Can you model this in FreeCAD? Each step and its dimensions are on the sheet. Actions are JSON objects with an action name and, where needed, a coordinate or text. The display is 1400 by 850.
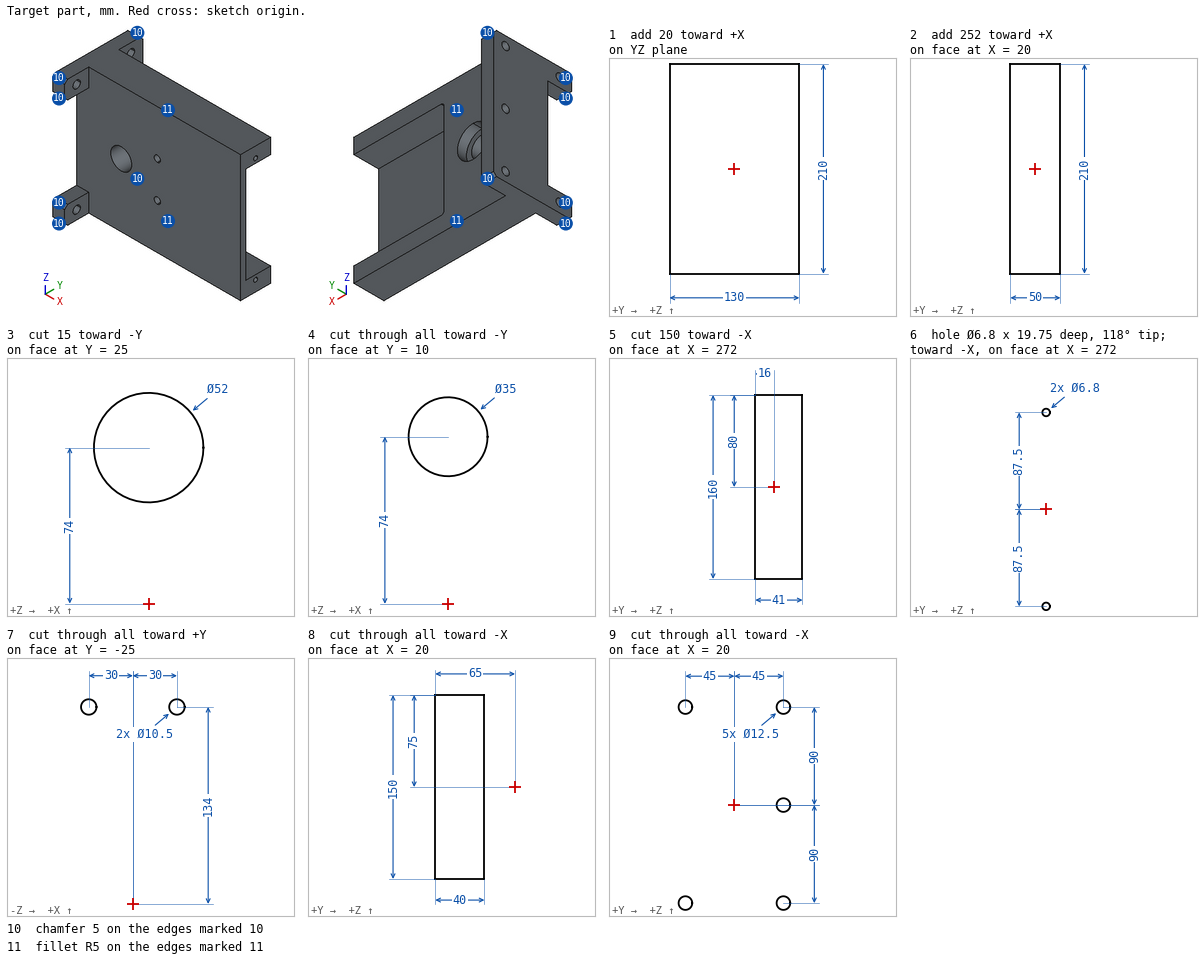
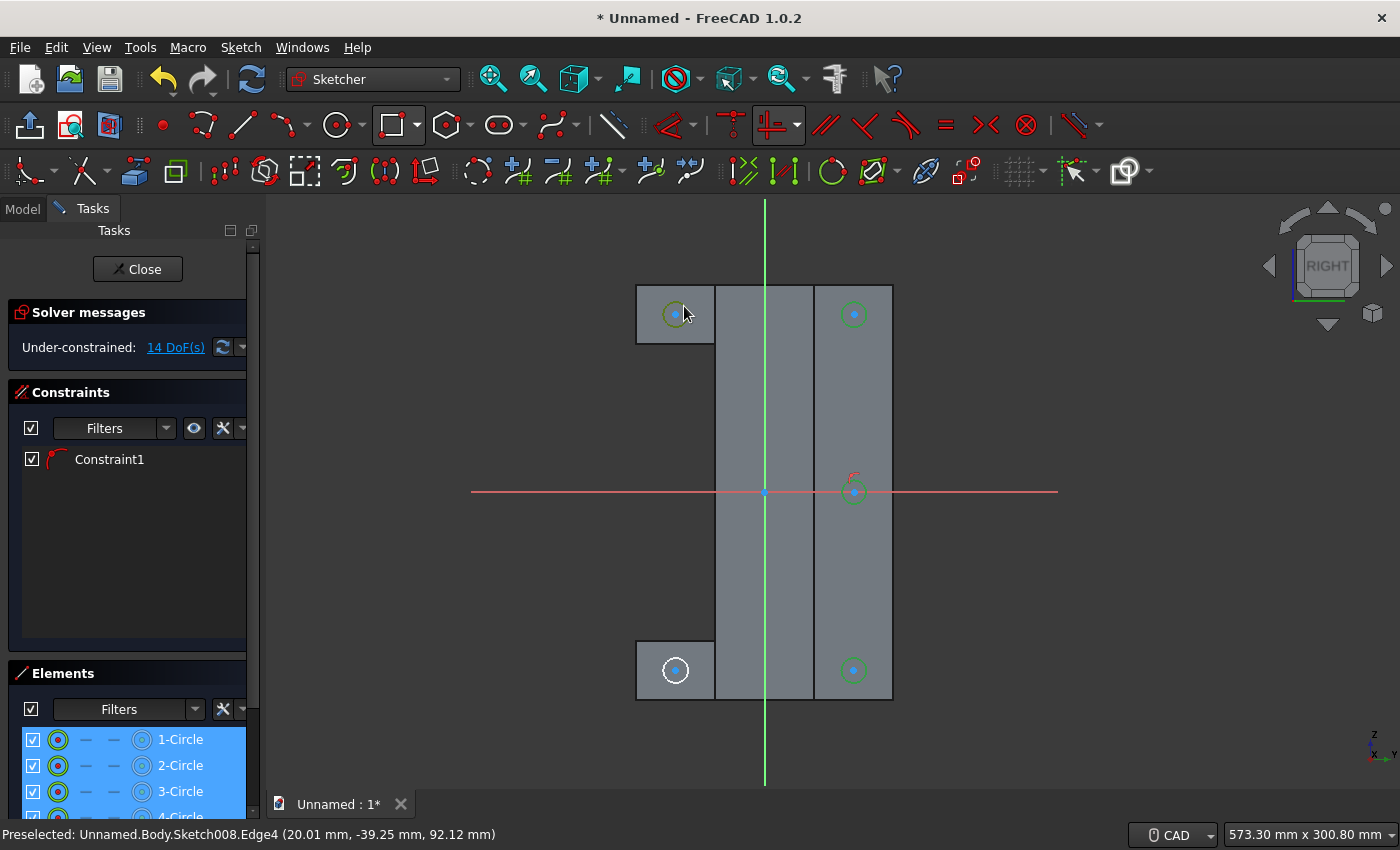
{"action": "left_click", "coordinate": [684, 662]}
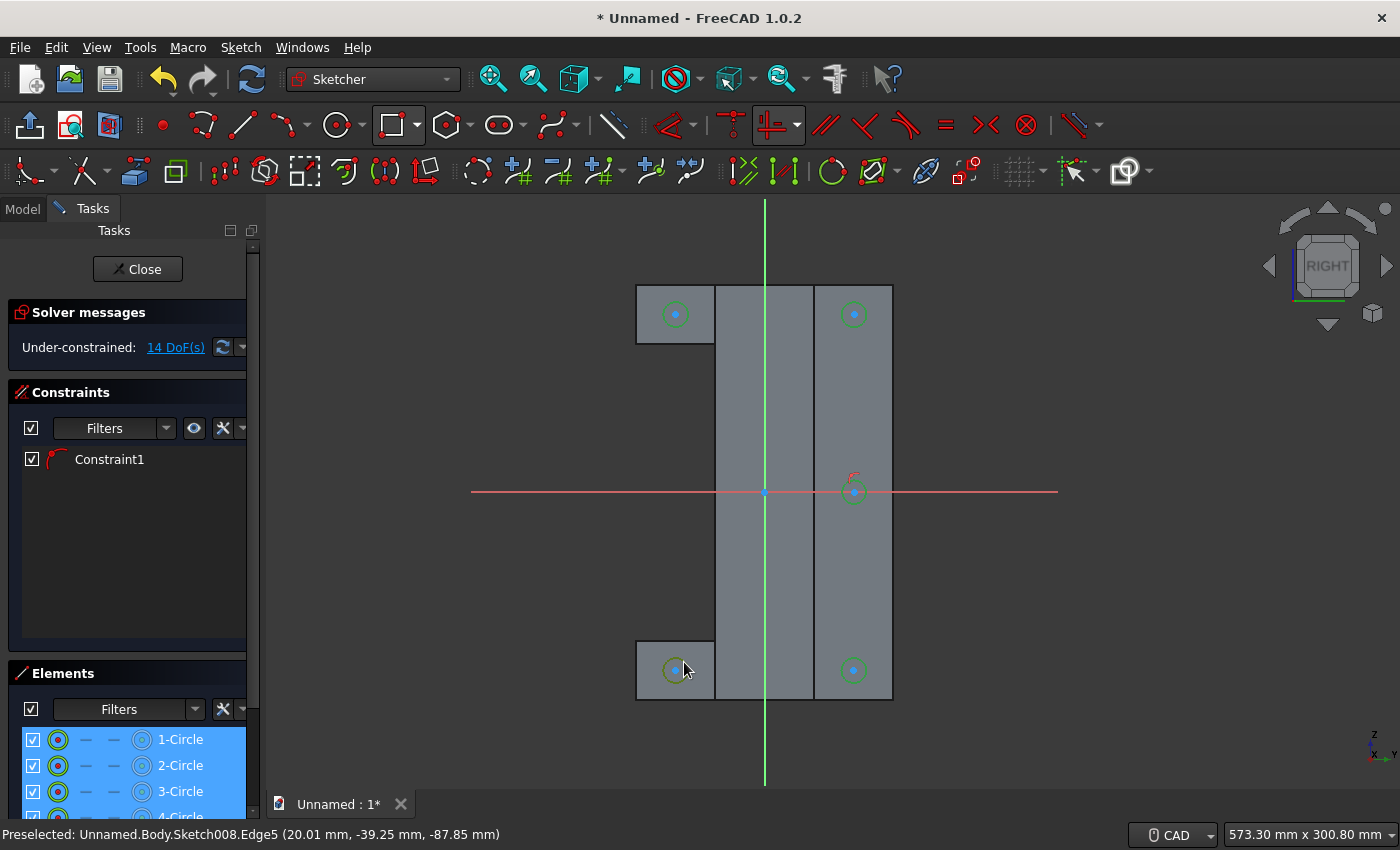
{"action": "left_click", "coordinate": [946, 126]}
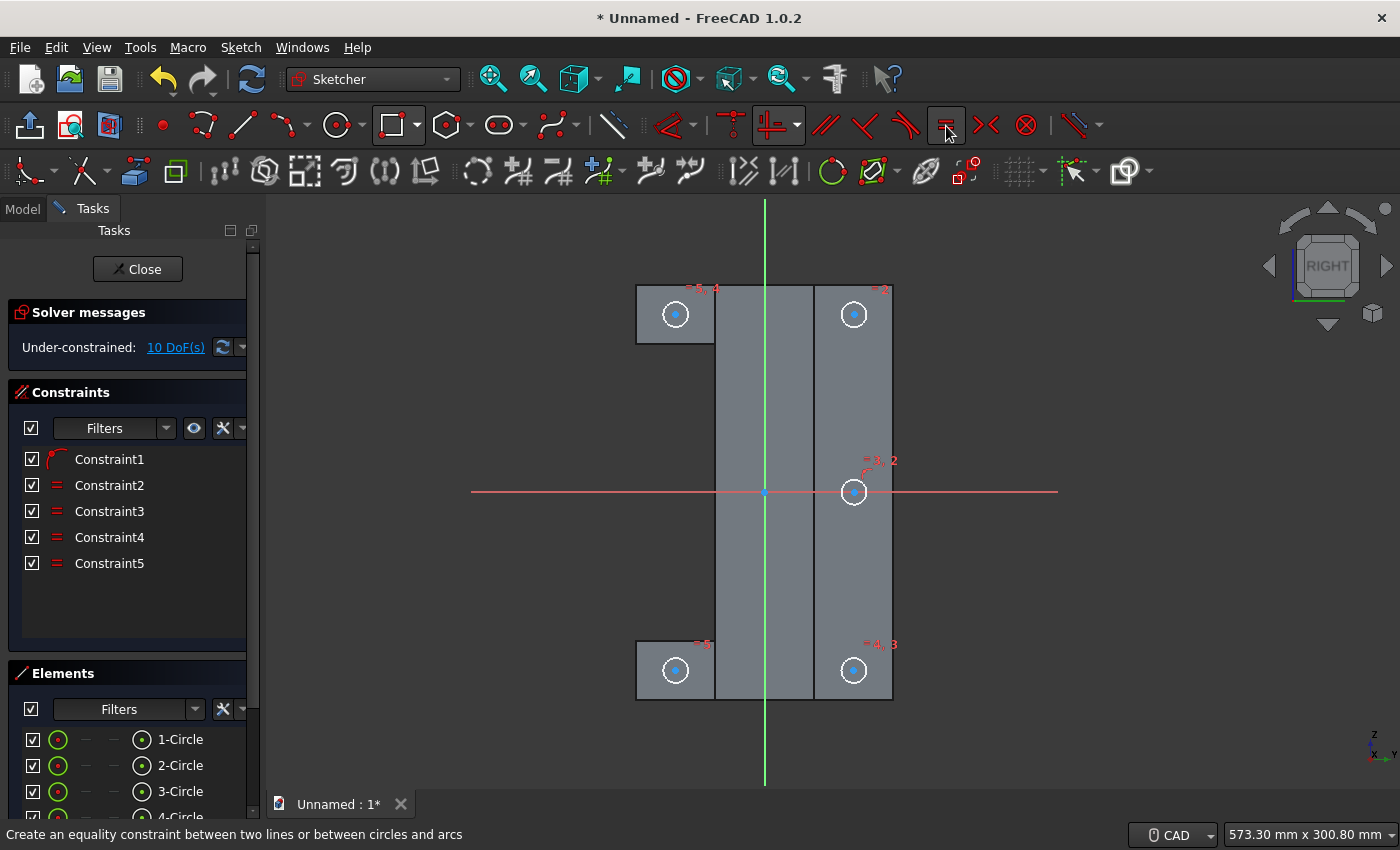
{"action": "left_click", "coordinate": [854, 315]}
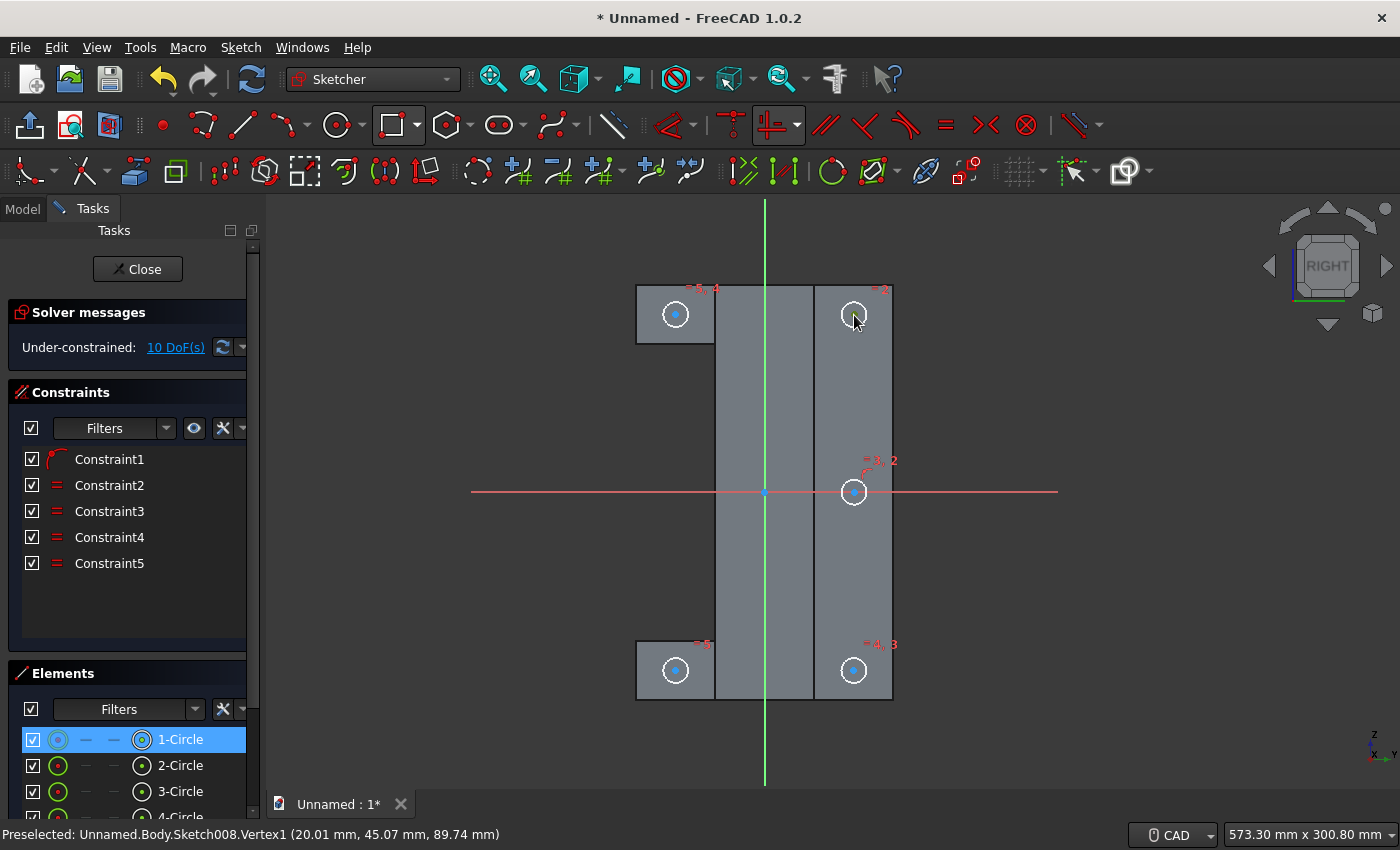
{"action": "left_click", "coordinate": [854, 492]}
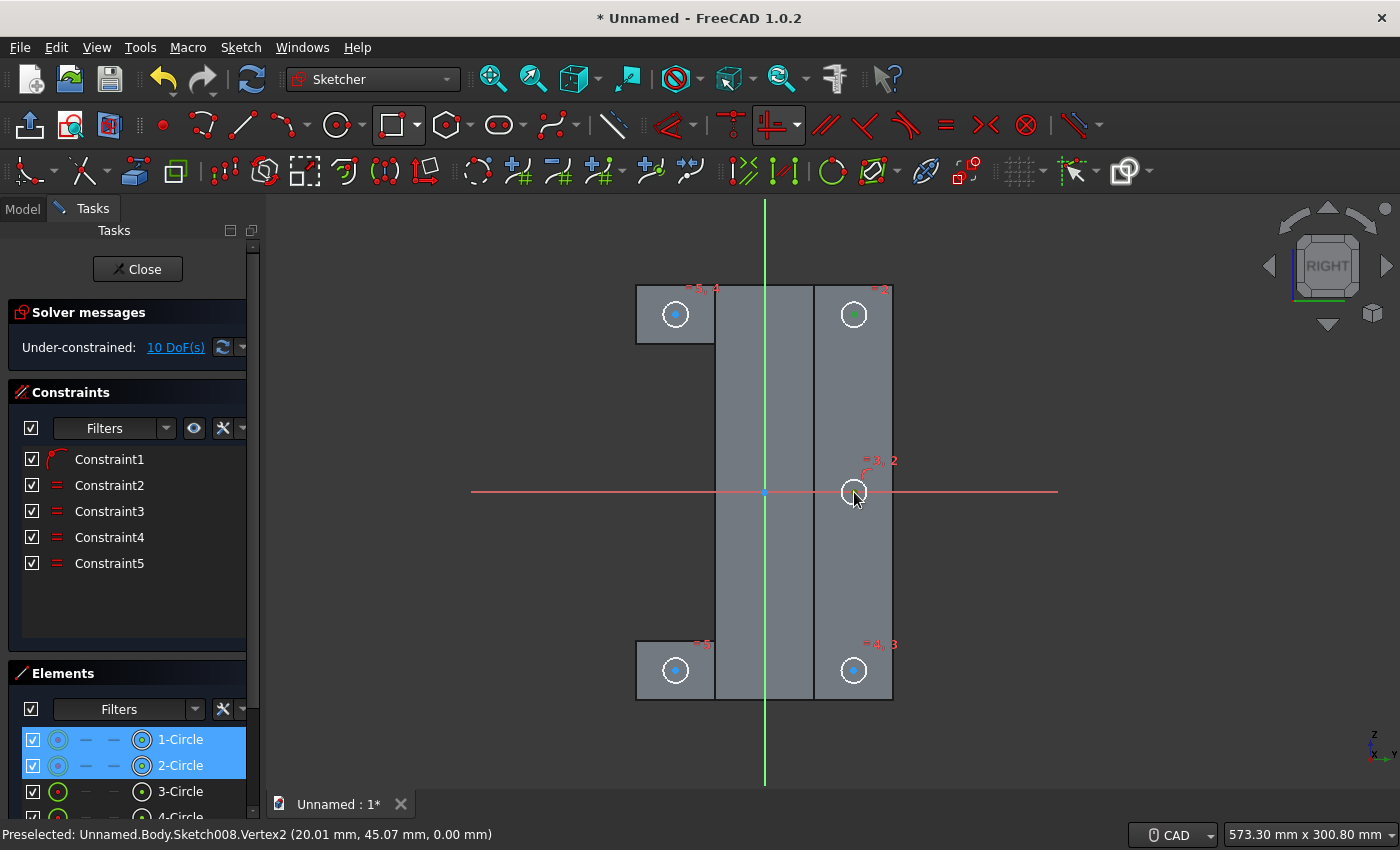
{"action": "key", "text": "v"}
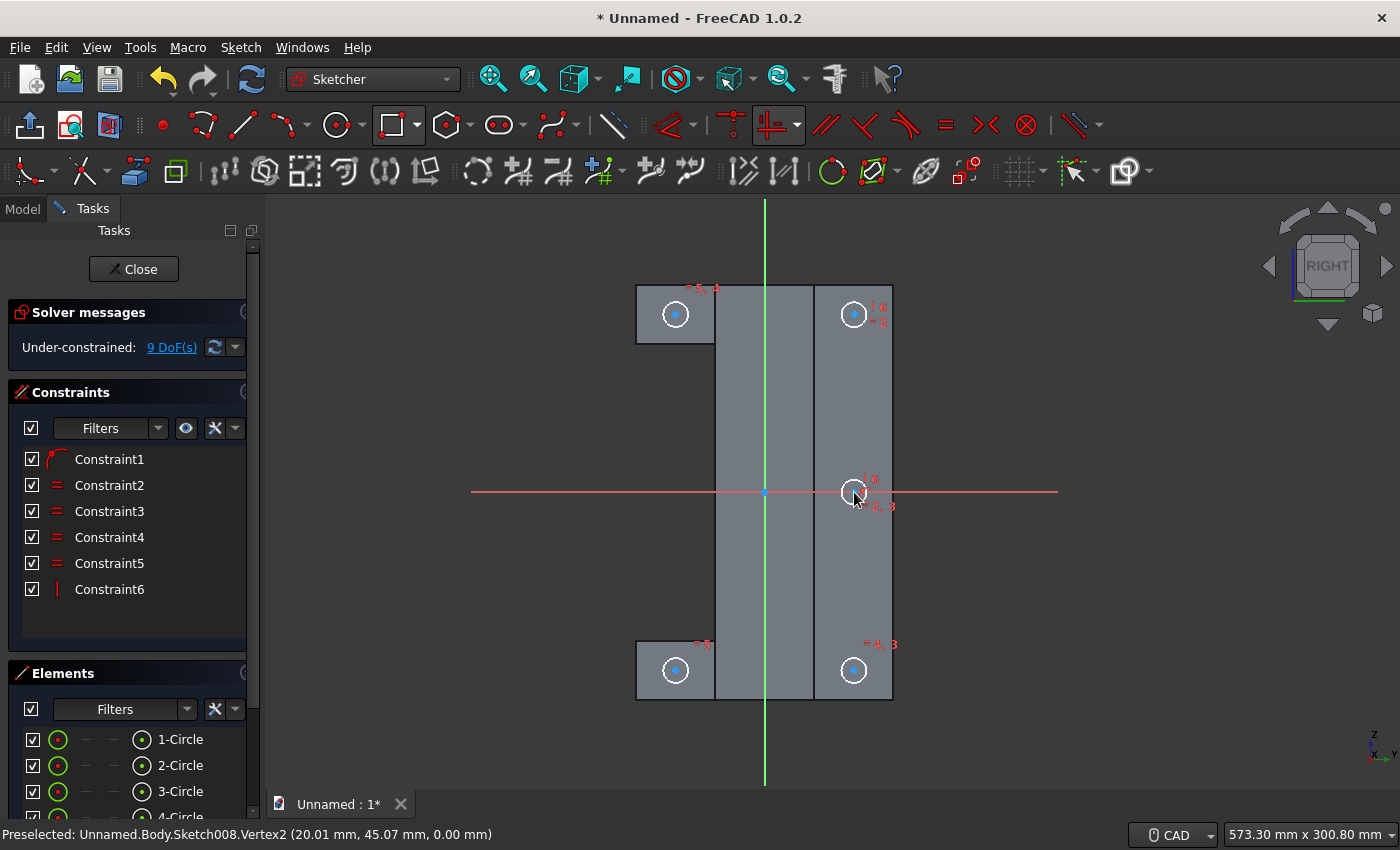
{"action": "left_click", "coordinate": [854, 492]}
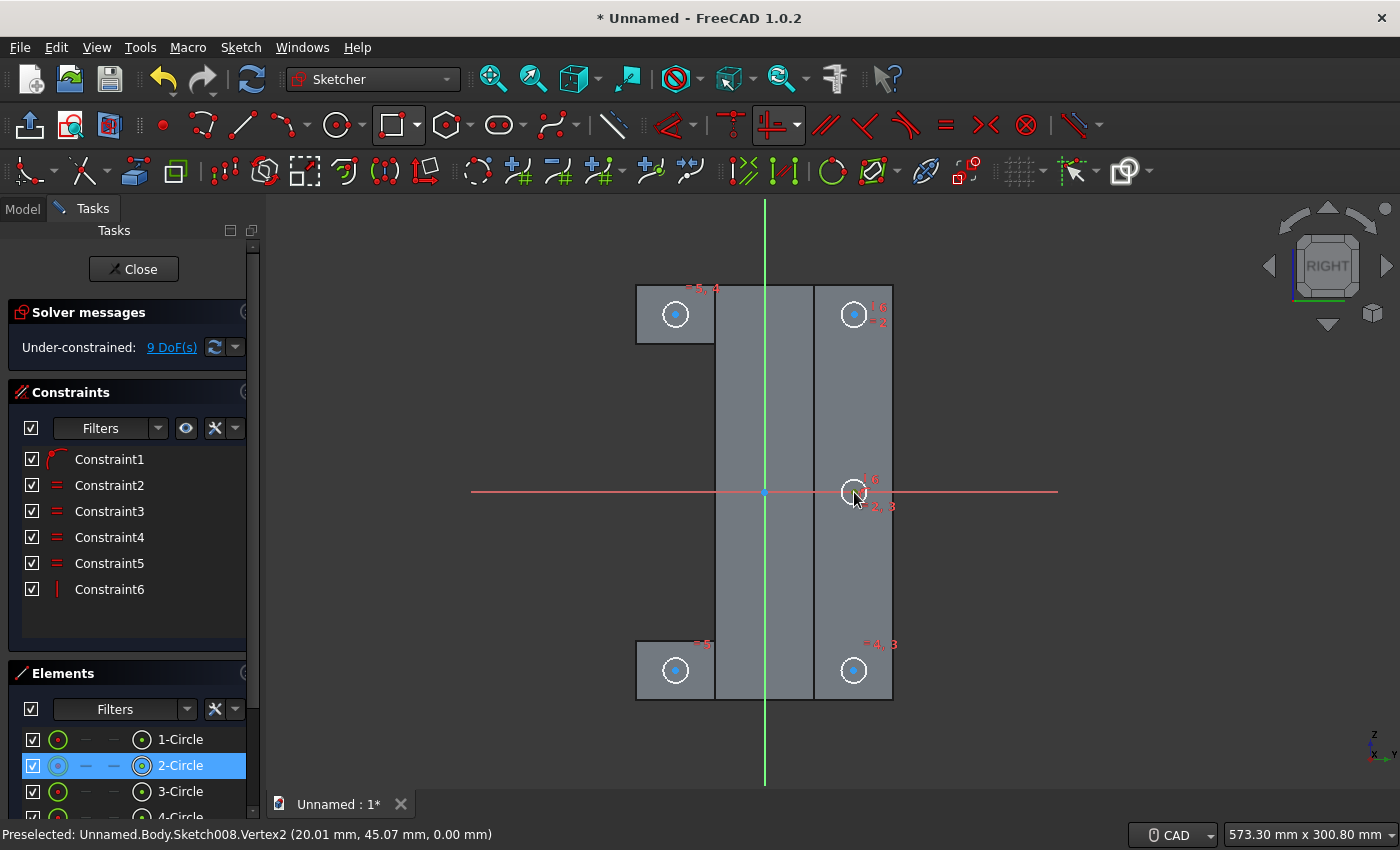
{"action": "left_click", "coordinate": [854, 671]}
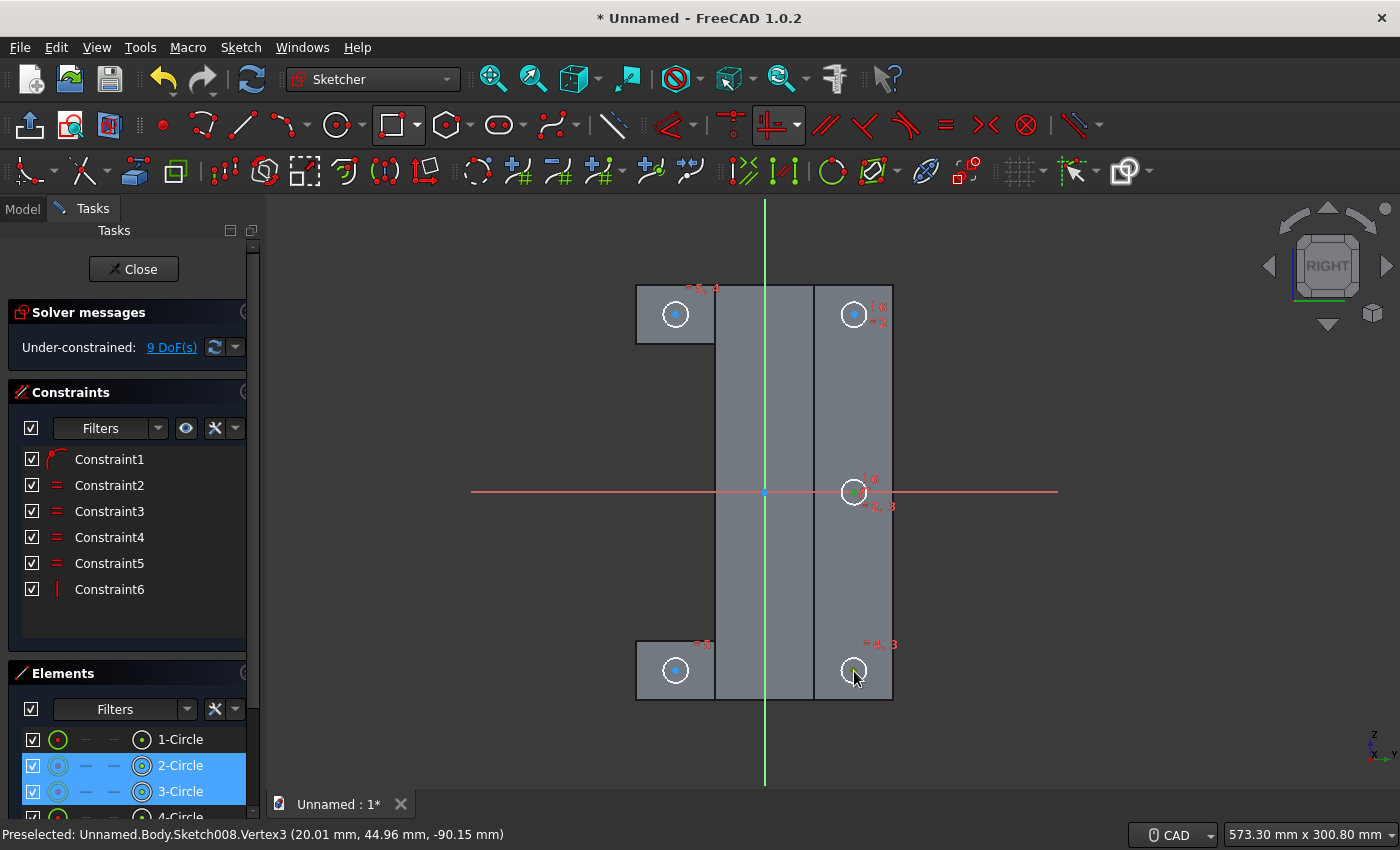
{"action": "left_click", "coordinate": [800, 126]}